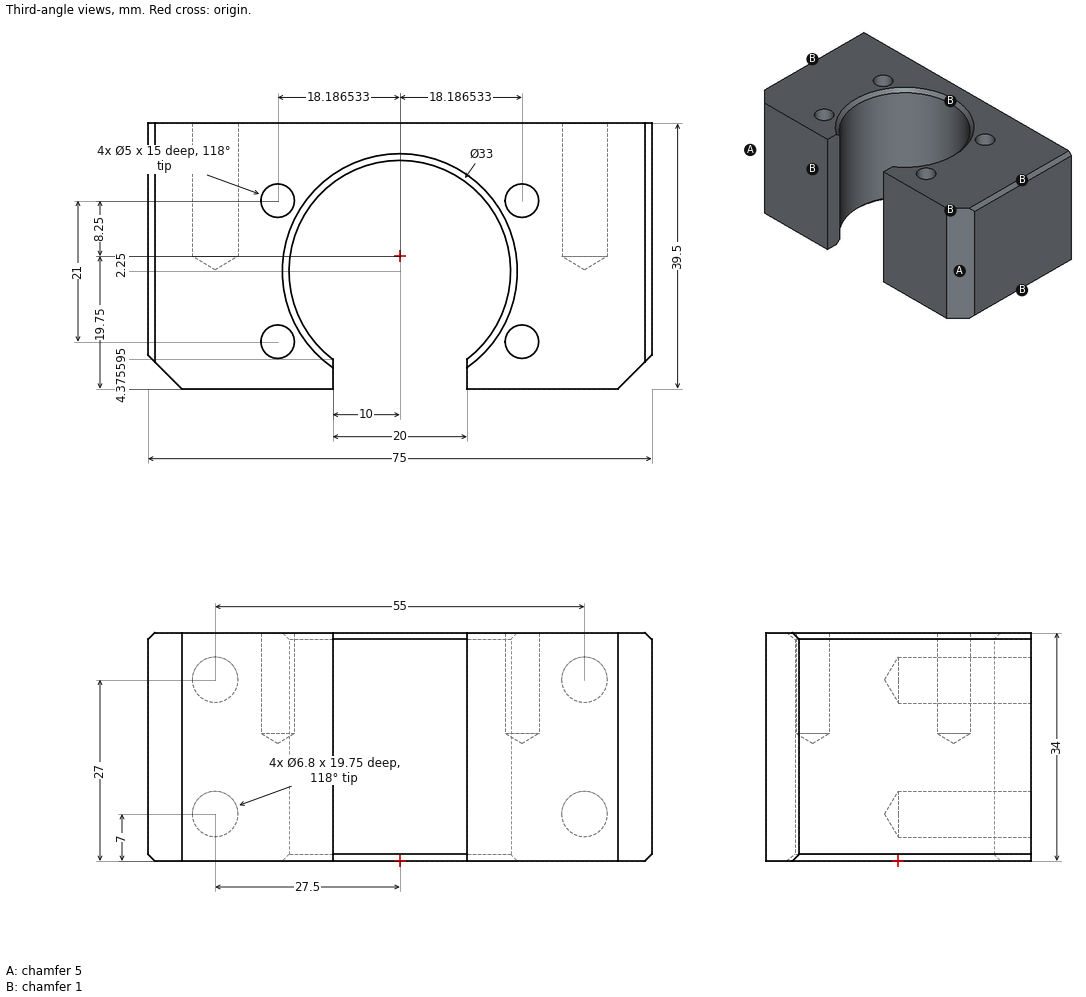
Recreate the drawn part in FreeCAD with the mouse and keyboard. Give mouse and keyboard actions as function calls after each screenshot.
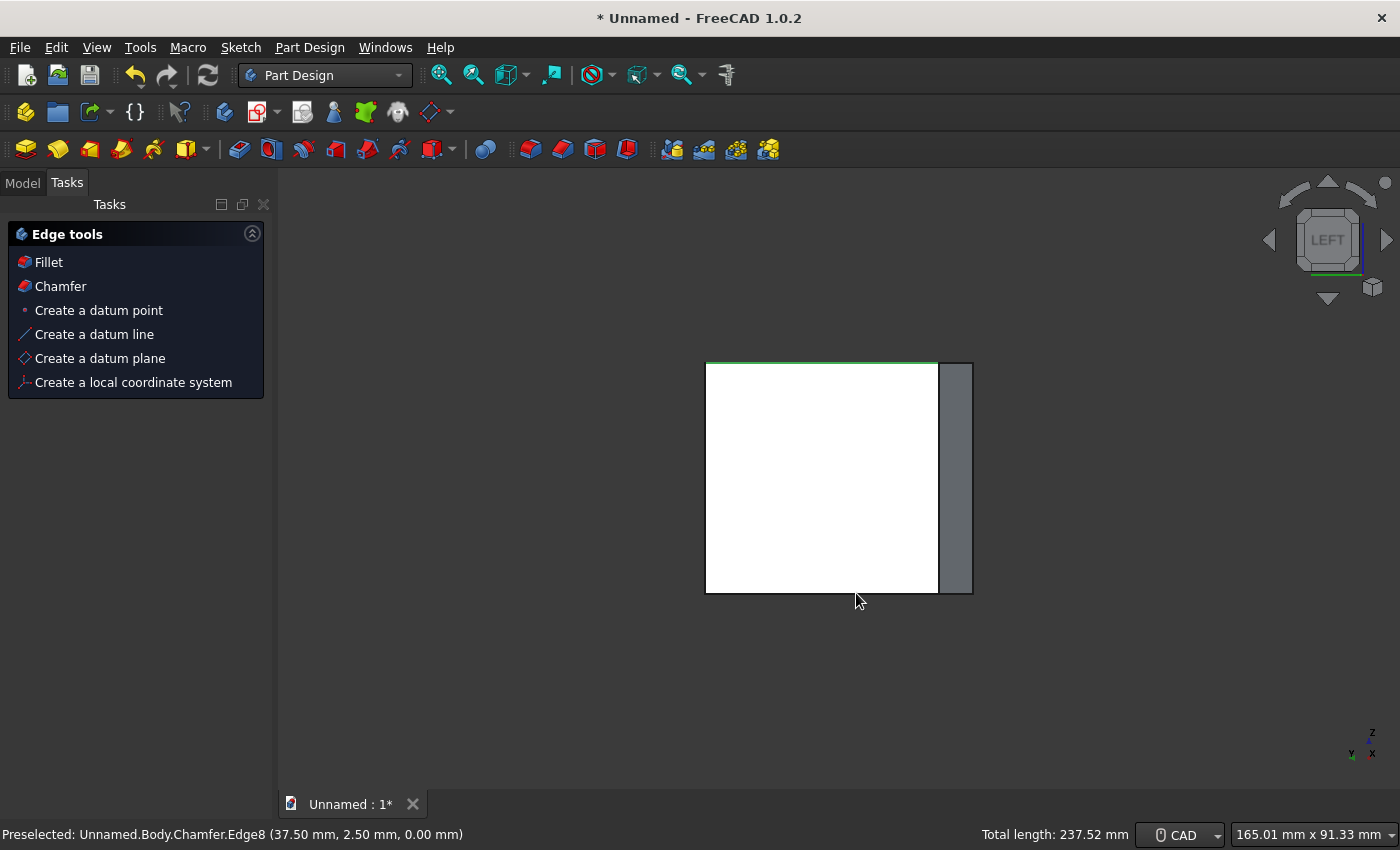
click(442, 76)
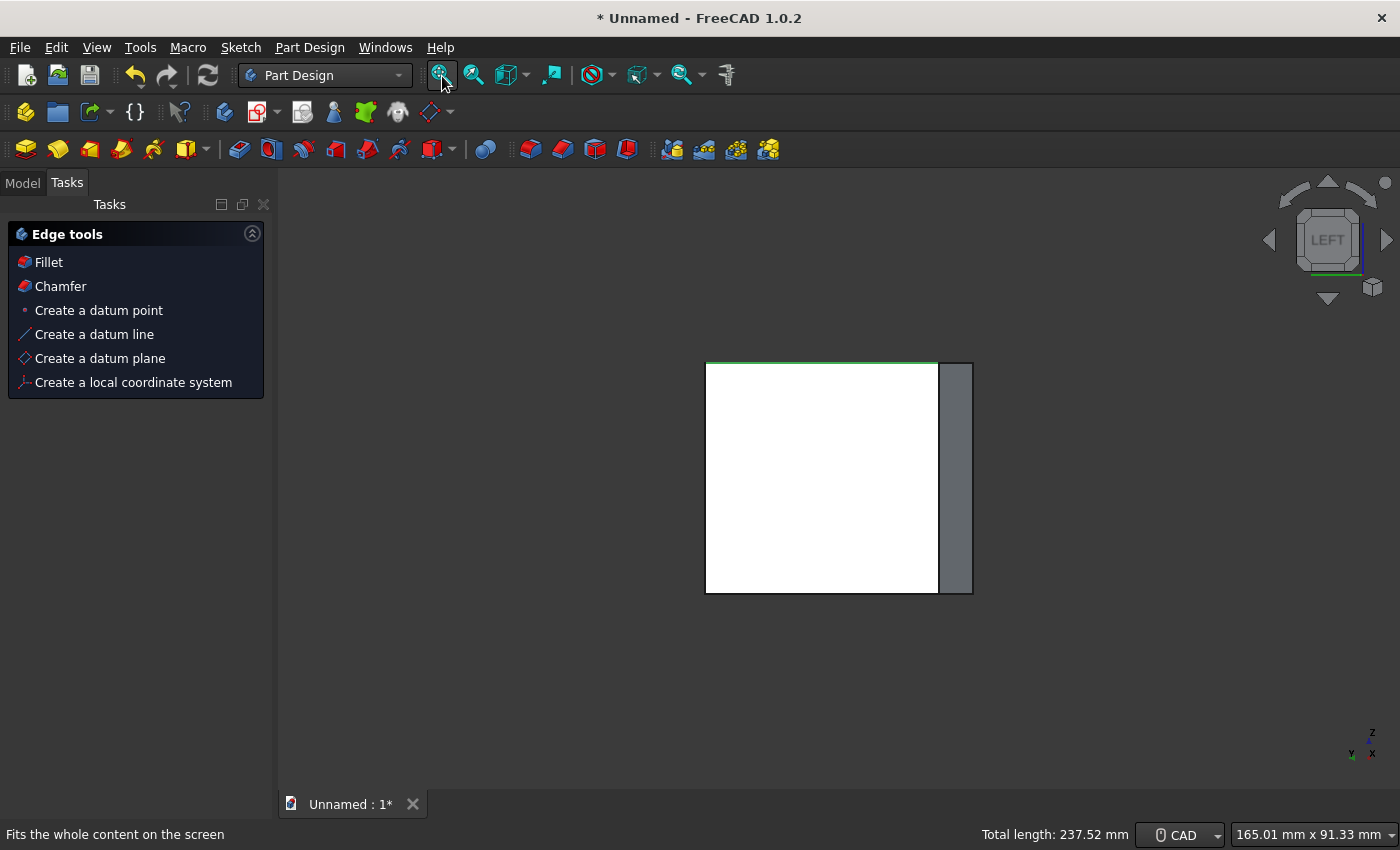
click(822, 593, ctrl)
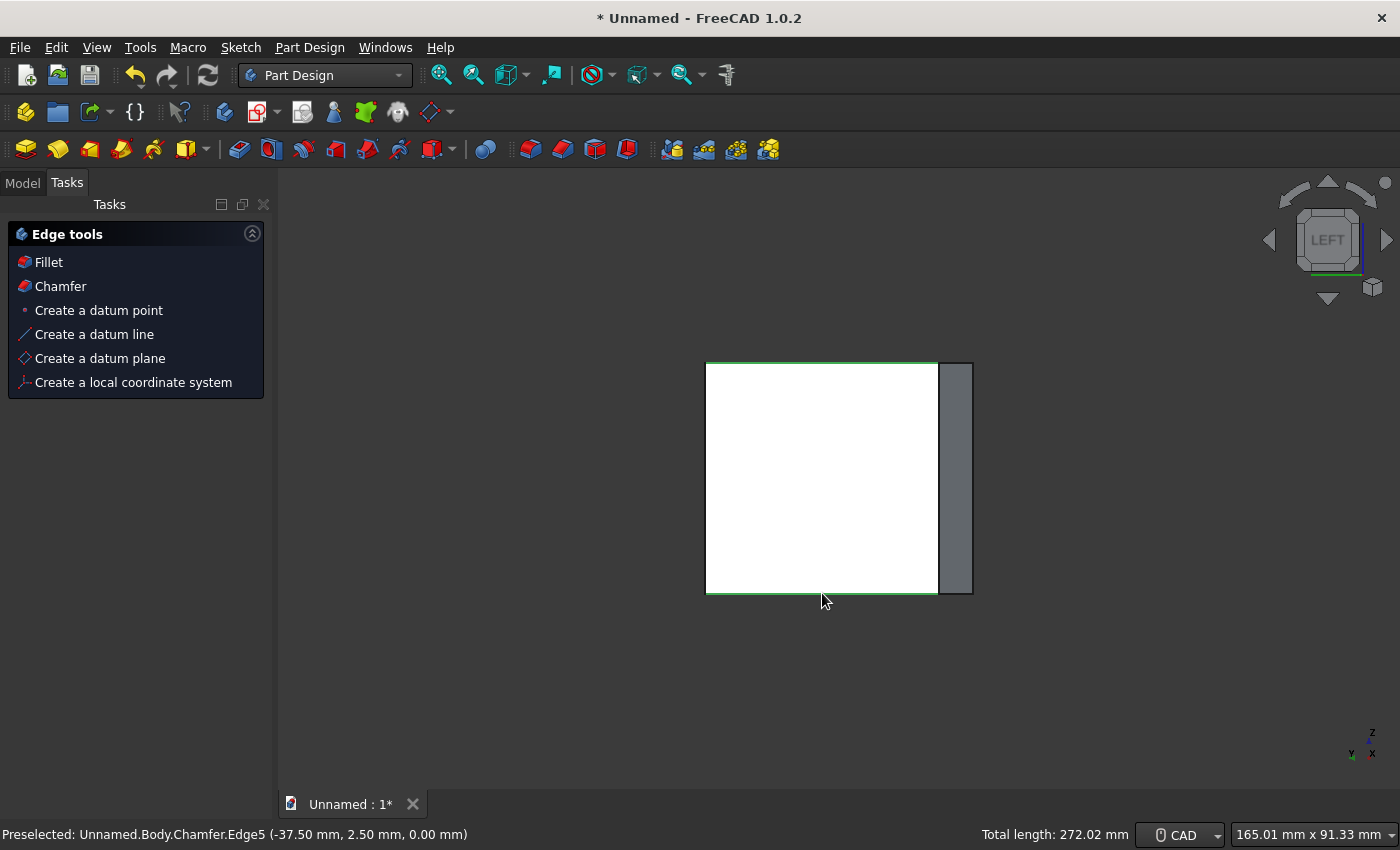
click(564, 150)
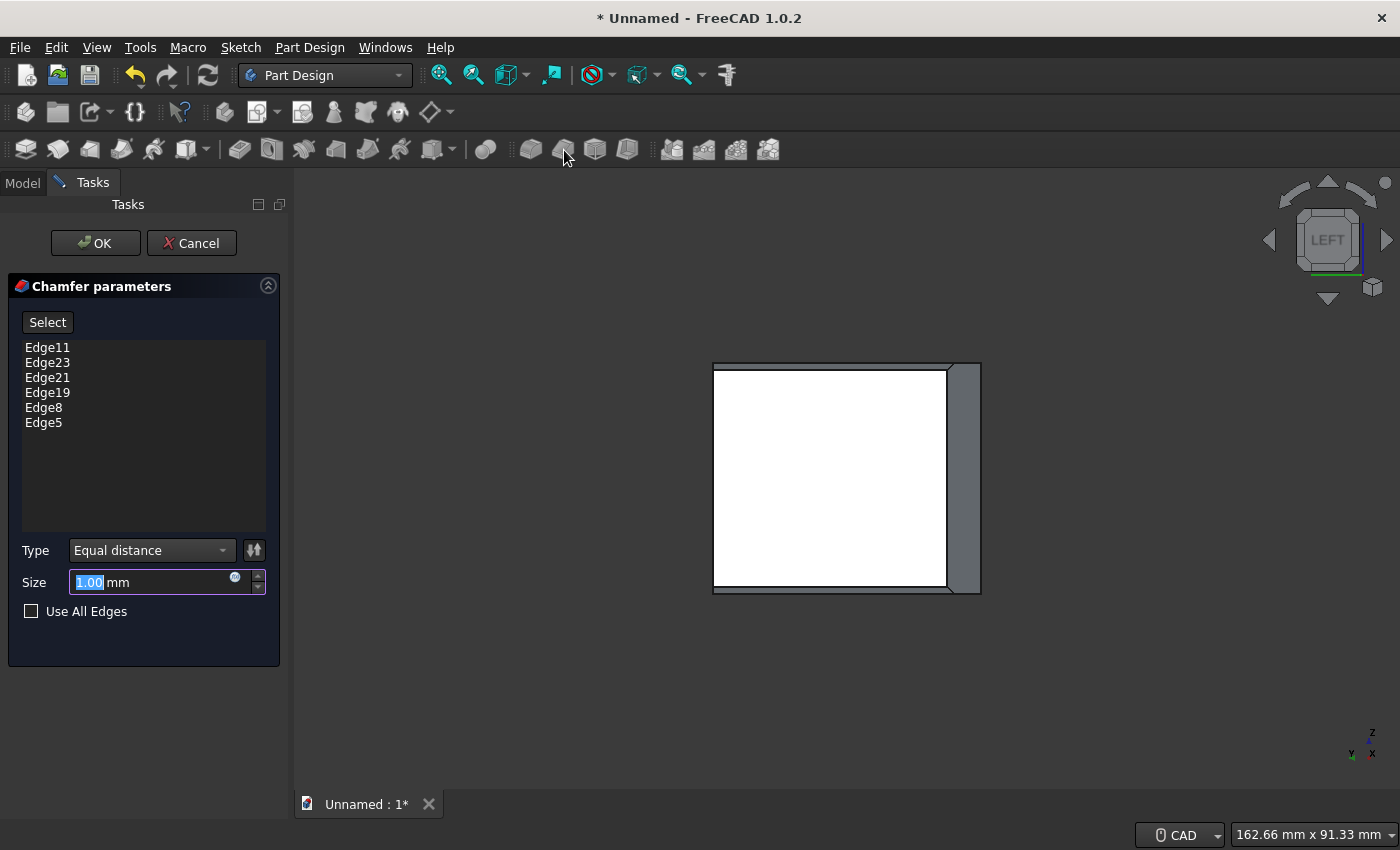
text(1)
key(Tab)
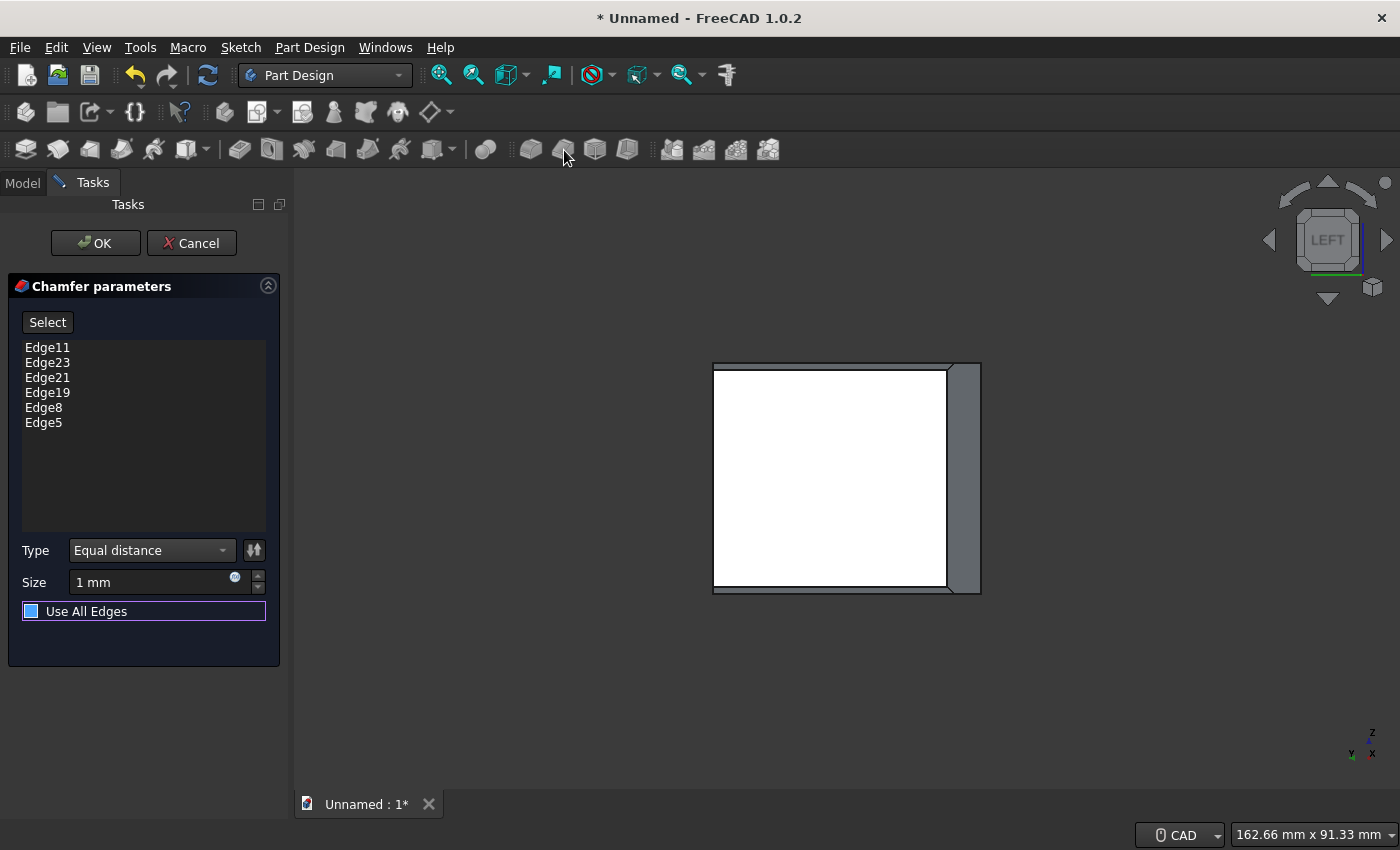
click(96, 243)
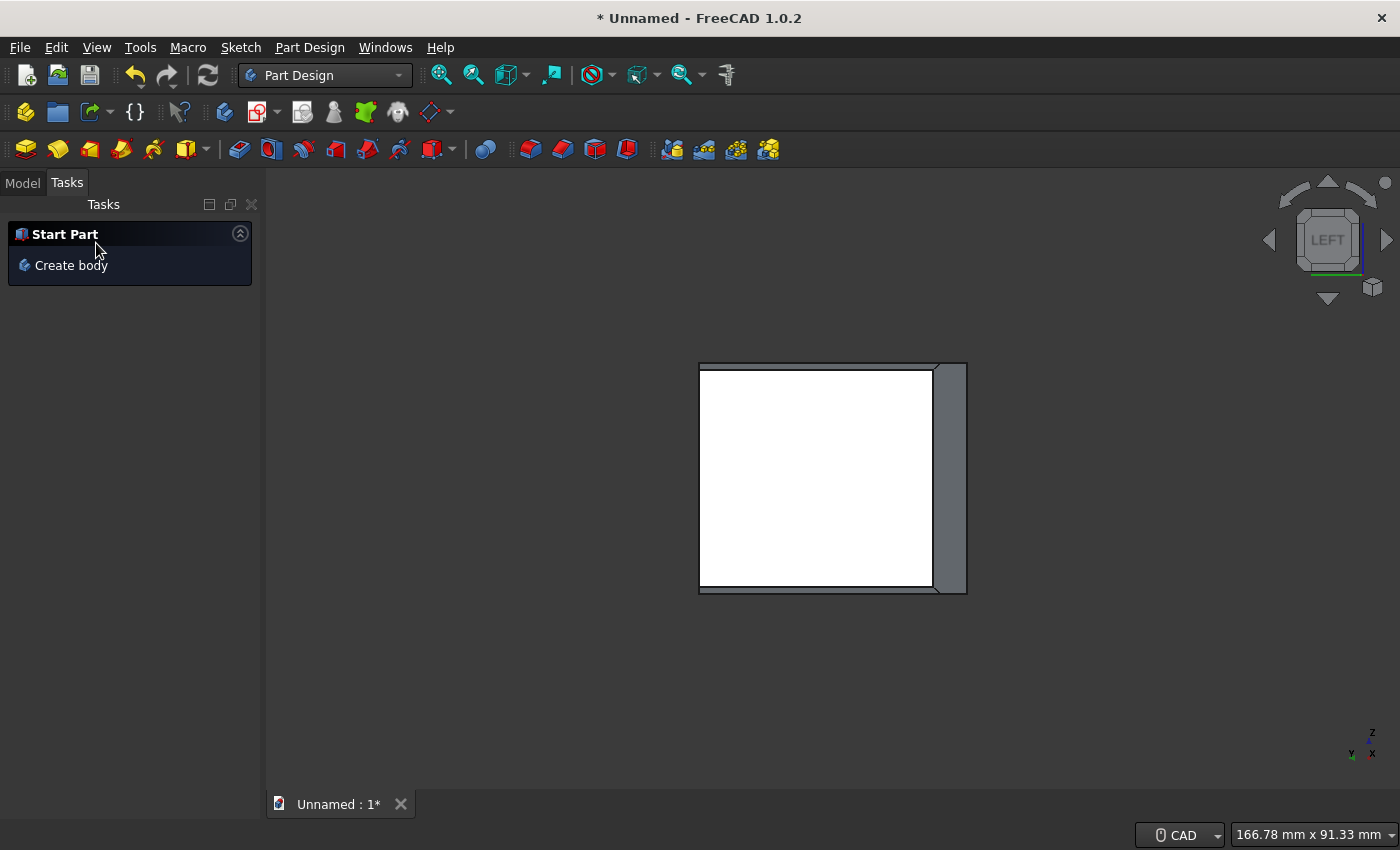
click(442, 76)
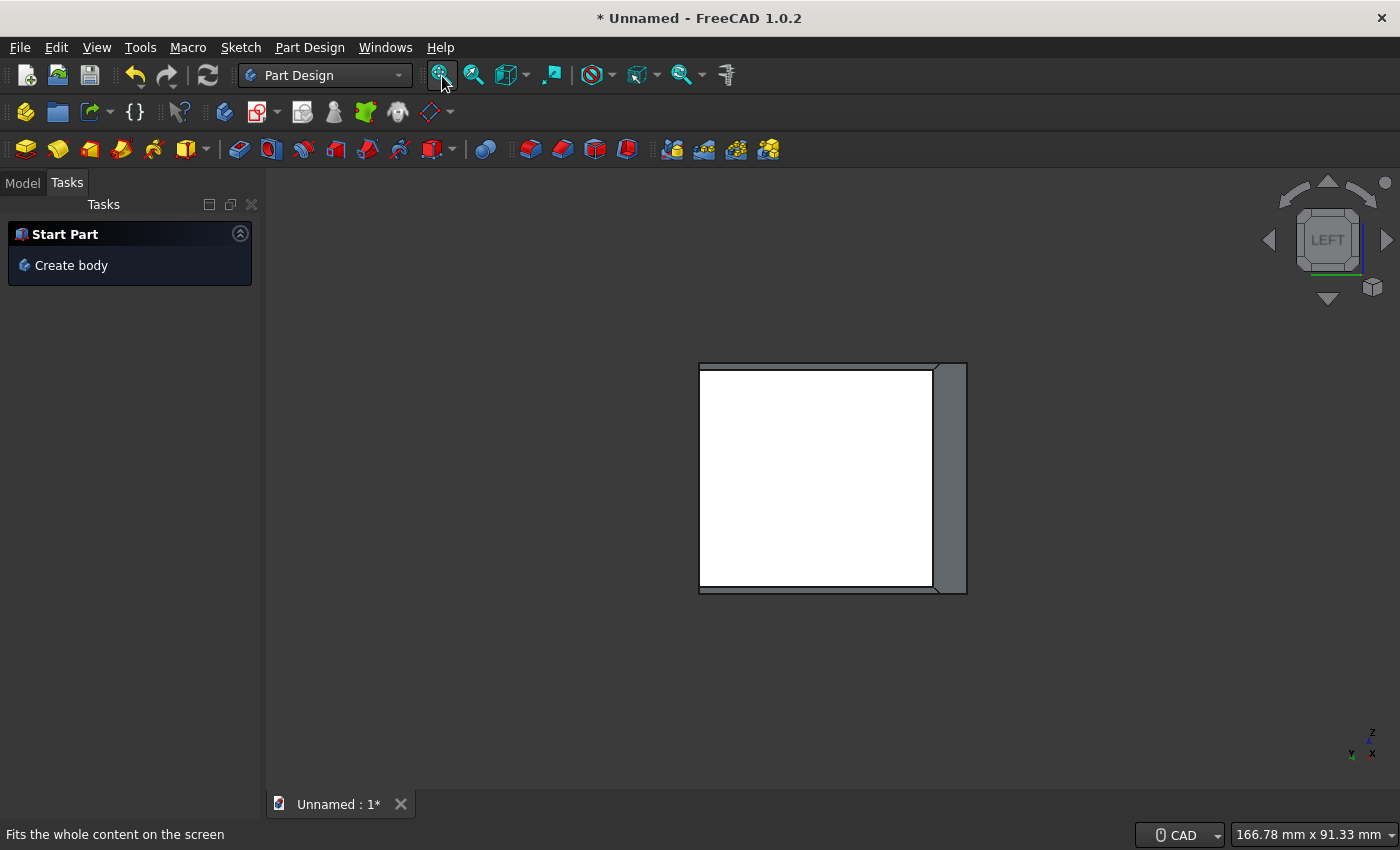
key(0)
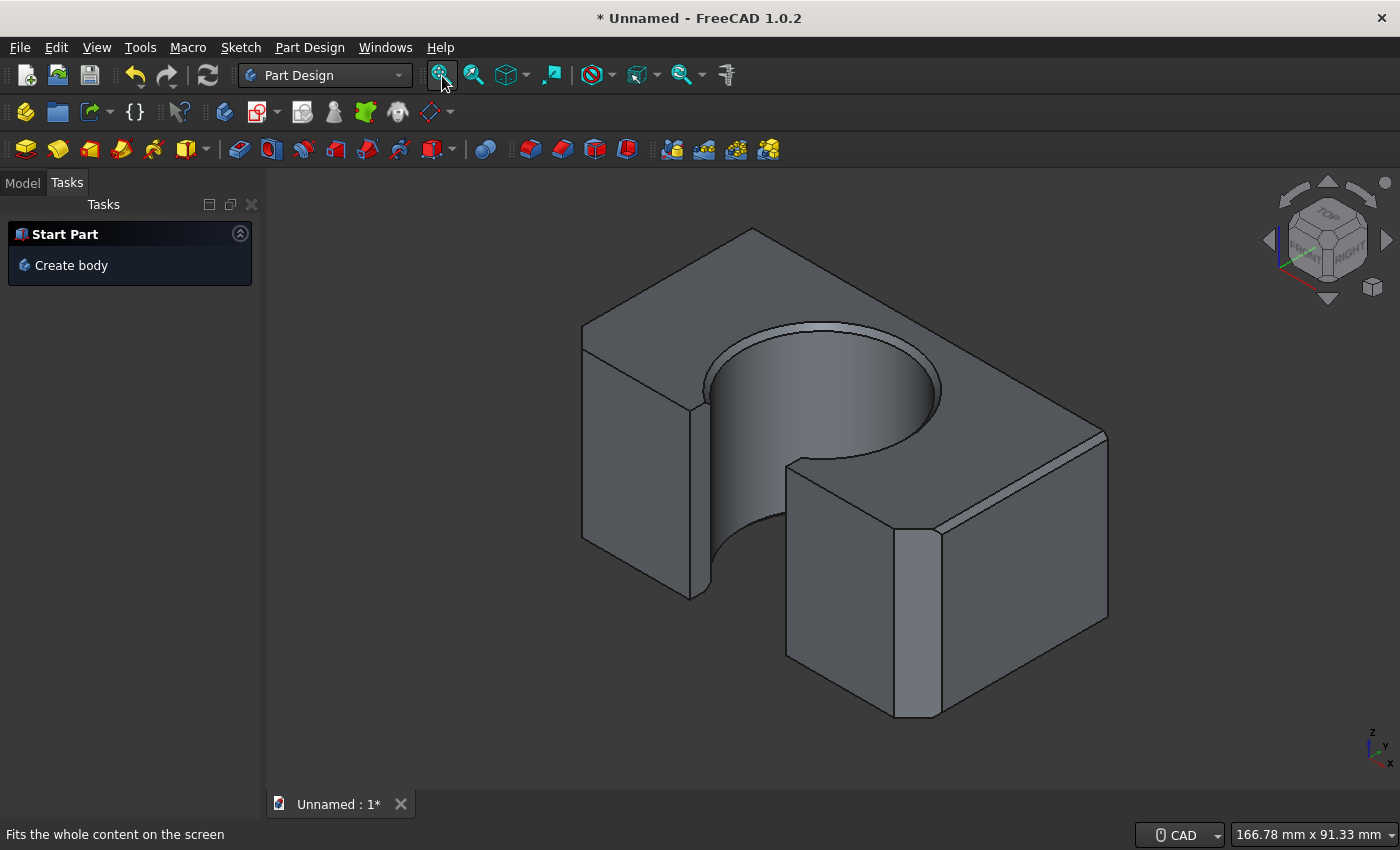
click(787, 294)